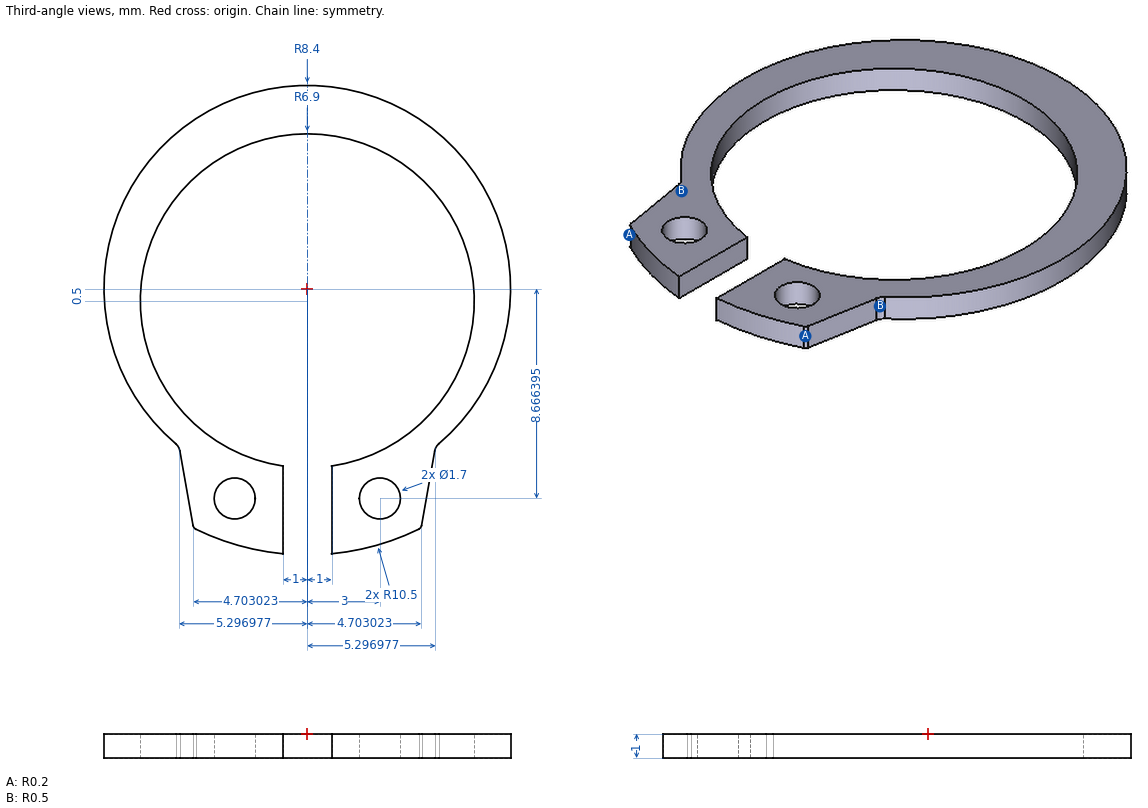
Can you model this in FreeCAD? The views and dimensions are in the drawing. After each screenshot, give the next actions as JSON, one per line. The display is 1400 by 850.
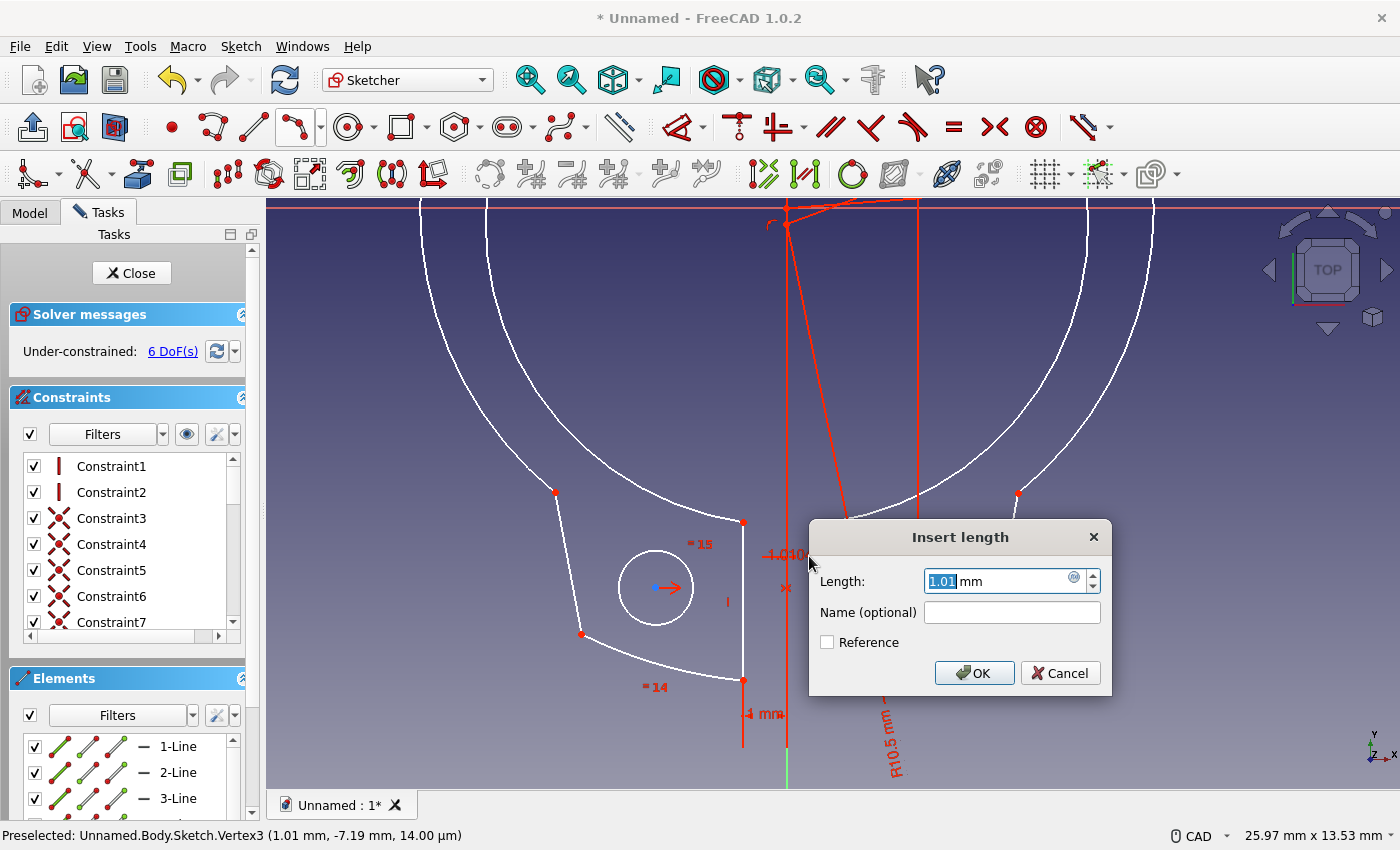
{"action": "type", "text": "1"}
{"action": "key", "text": "Return"}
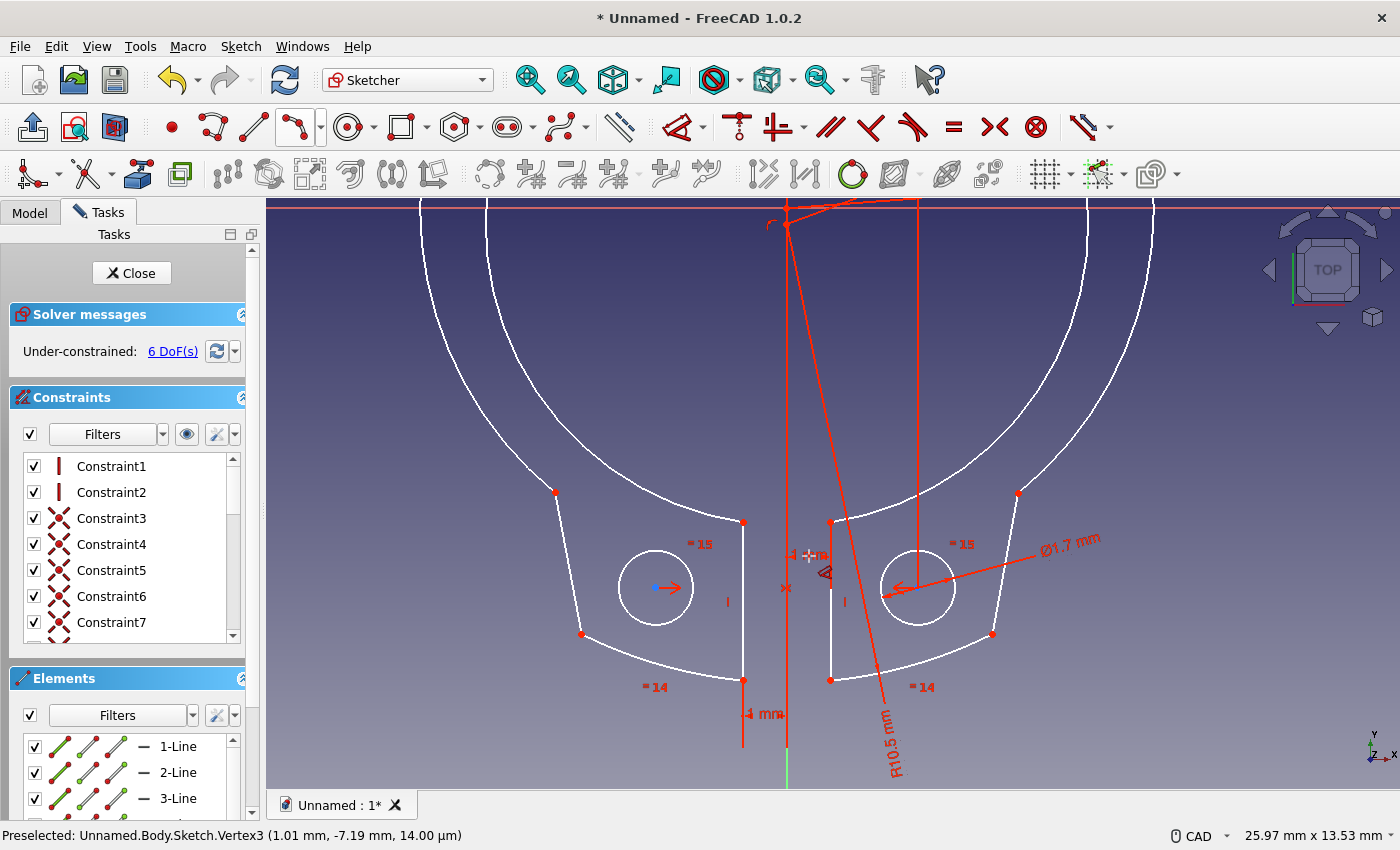
{"action": "scroll", "coordinate": [746, 681], "scroll_direction": "down", "scroll_amount": 4}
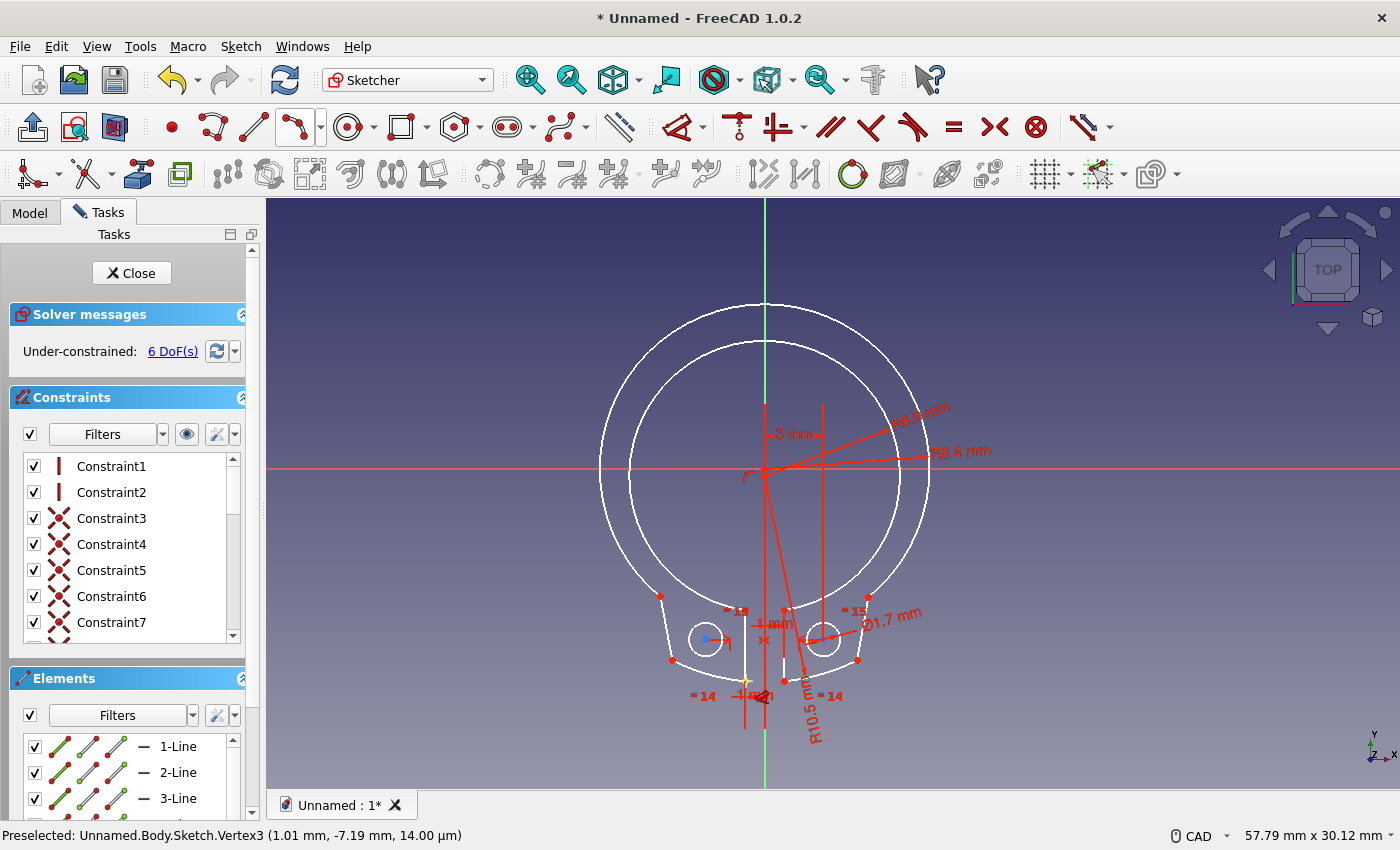
{"action": "scroll", "coordinate": [765, 476], "scroll_direction": "up", "scroll_amount": 7}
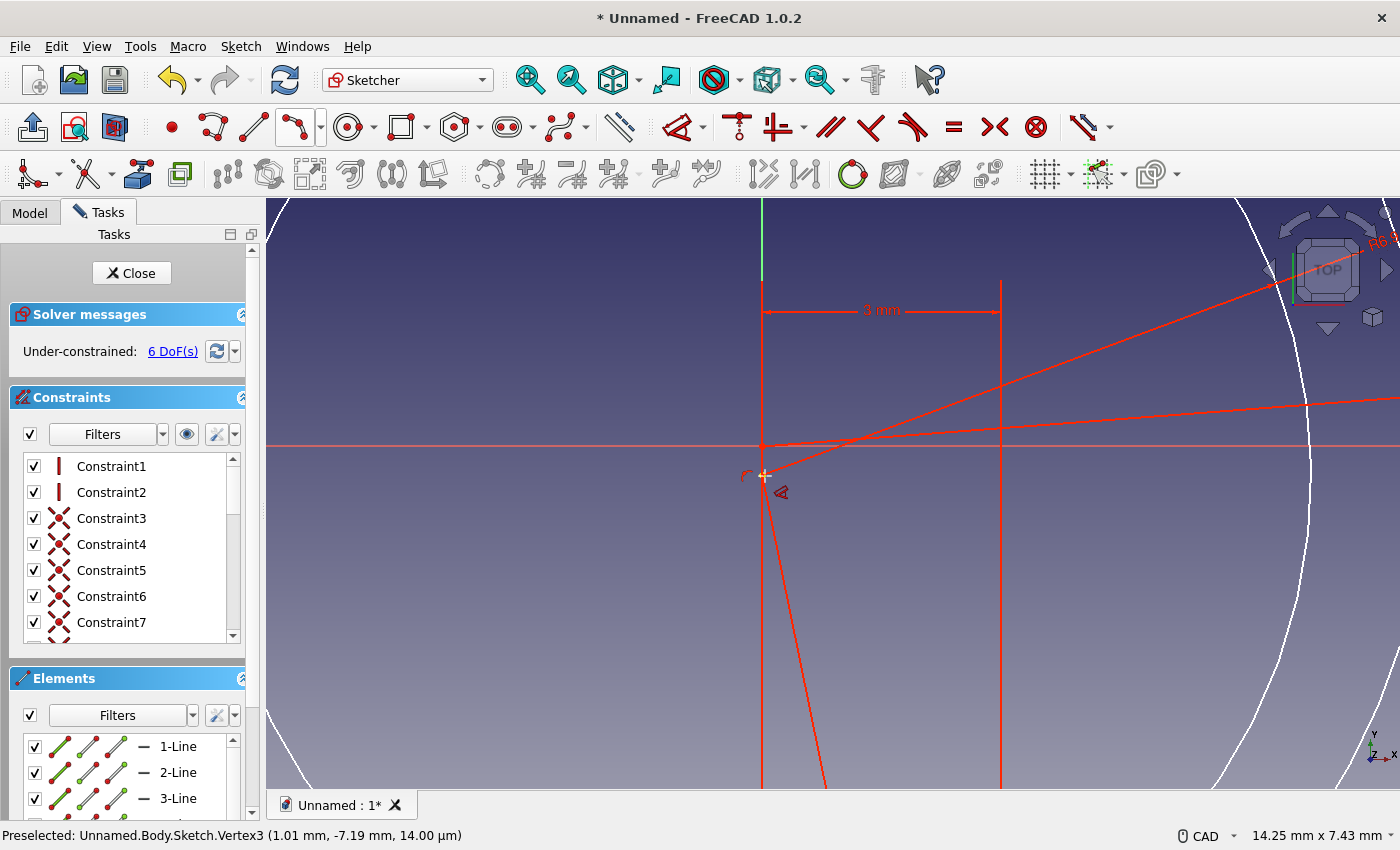
{"action": "left_click", "coordinate": [762, 475]}
{"action": "left_click", "coordinate": [796, 461]}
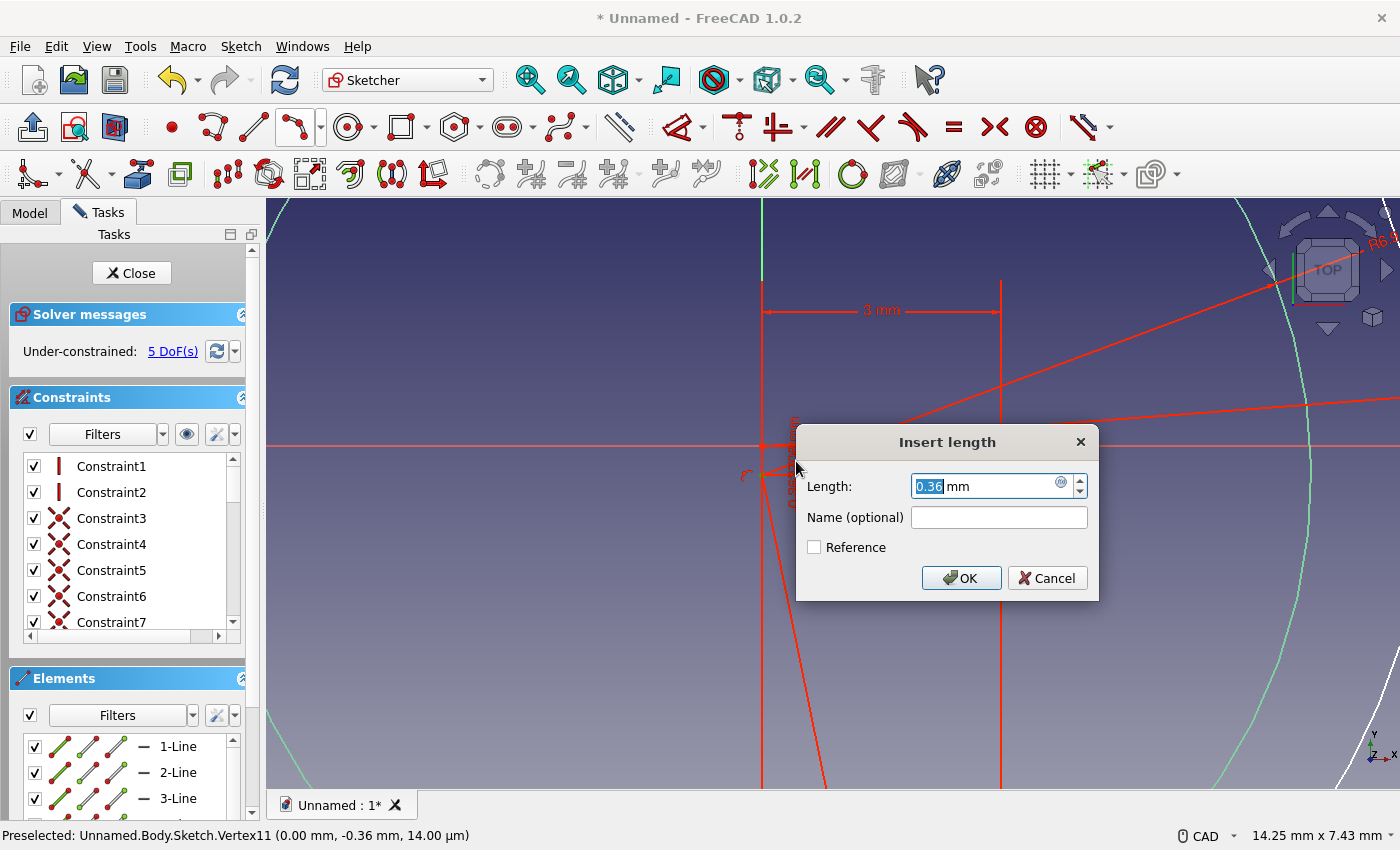
{"action": "type", "text": "0.5"}
{"action": "key", "text": "Return"}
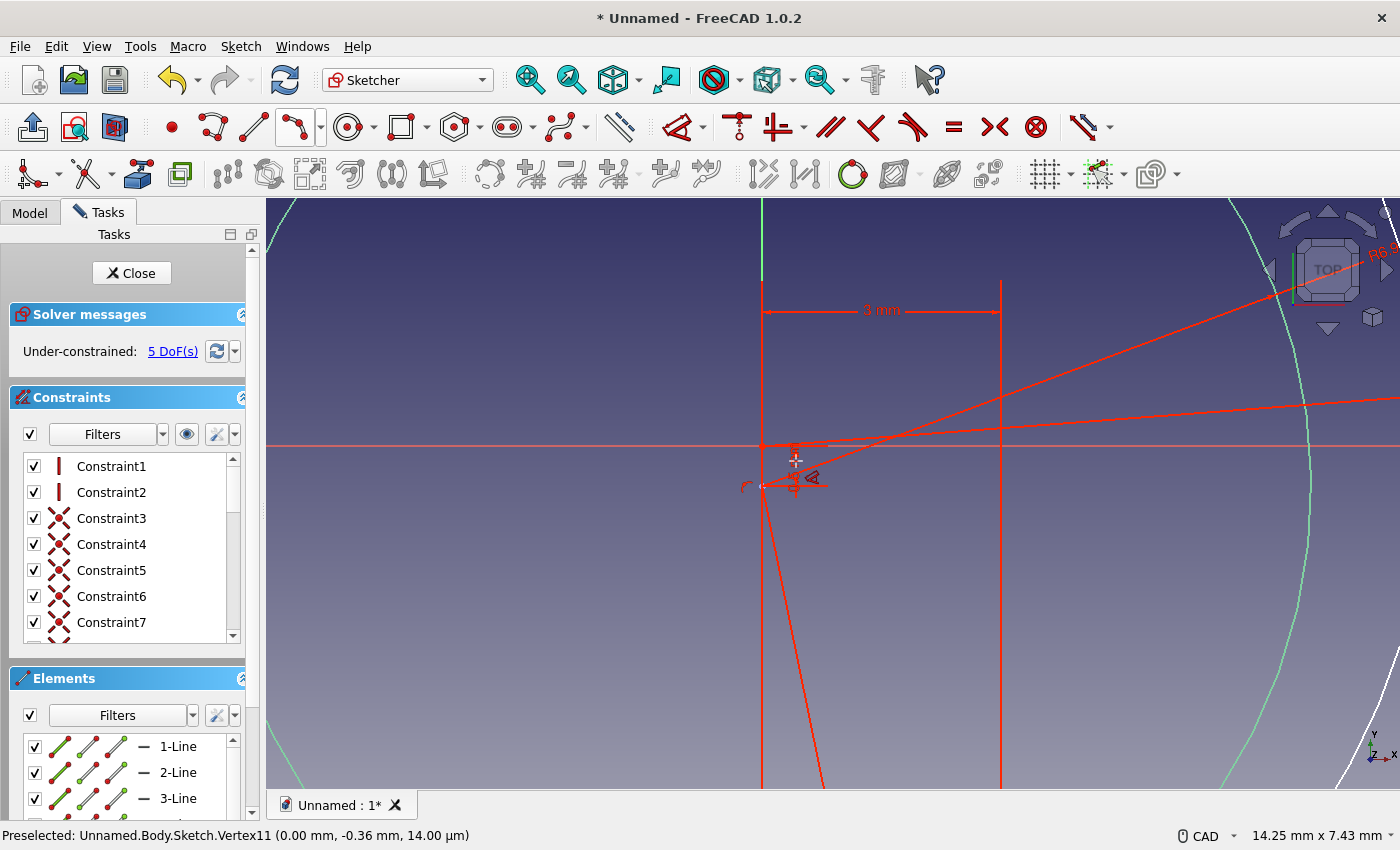
{"action": "scroll", "coordinate": [765, 476], "scroll_direction": "down", "scroll_amount": 7}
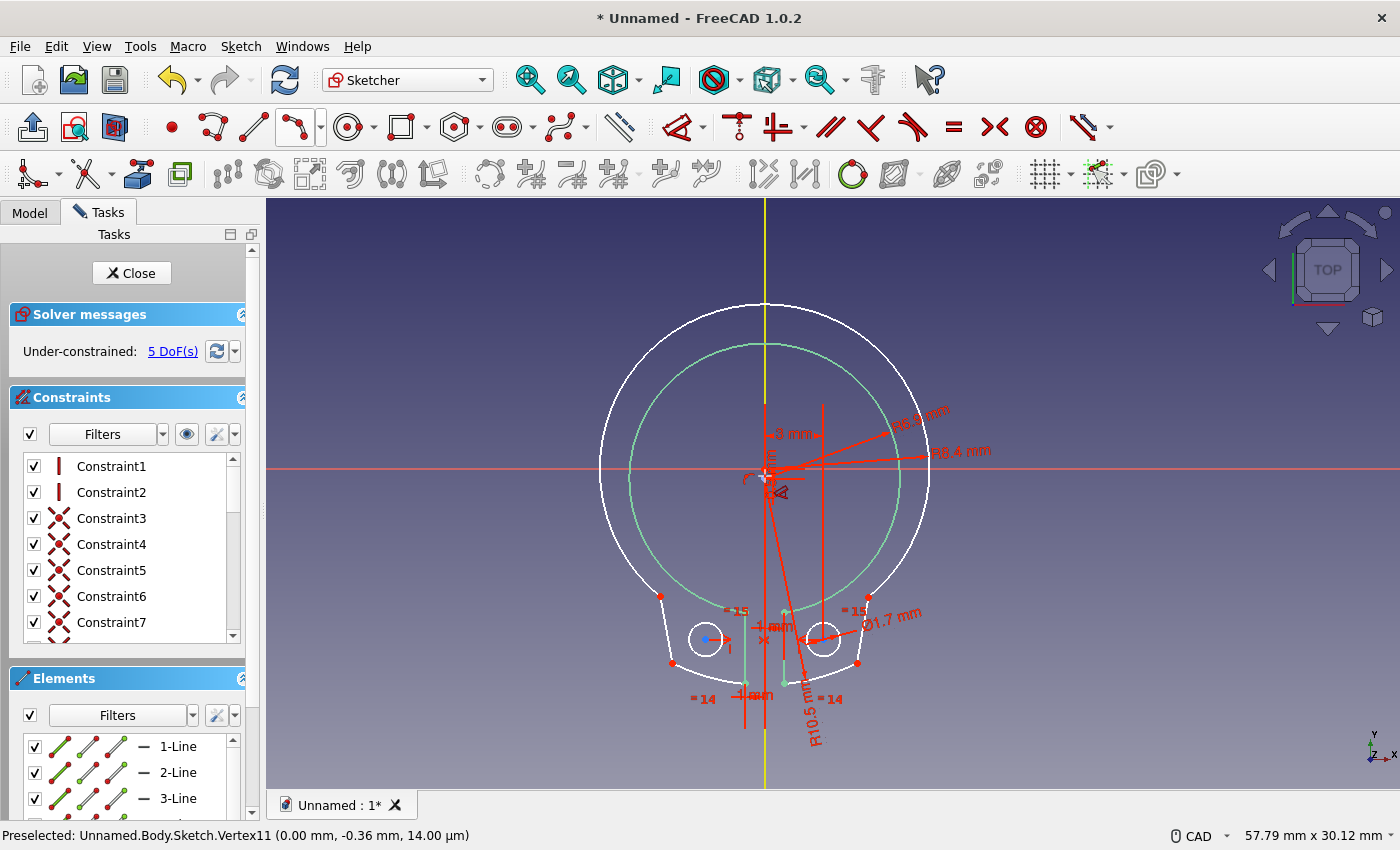
{"action": "left_click", "coordinate": [824, 640]}
{"action": "left_click", "coordinate": [858, 554]}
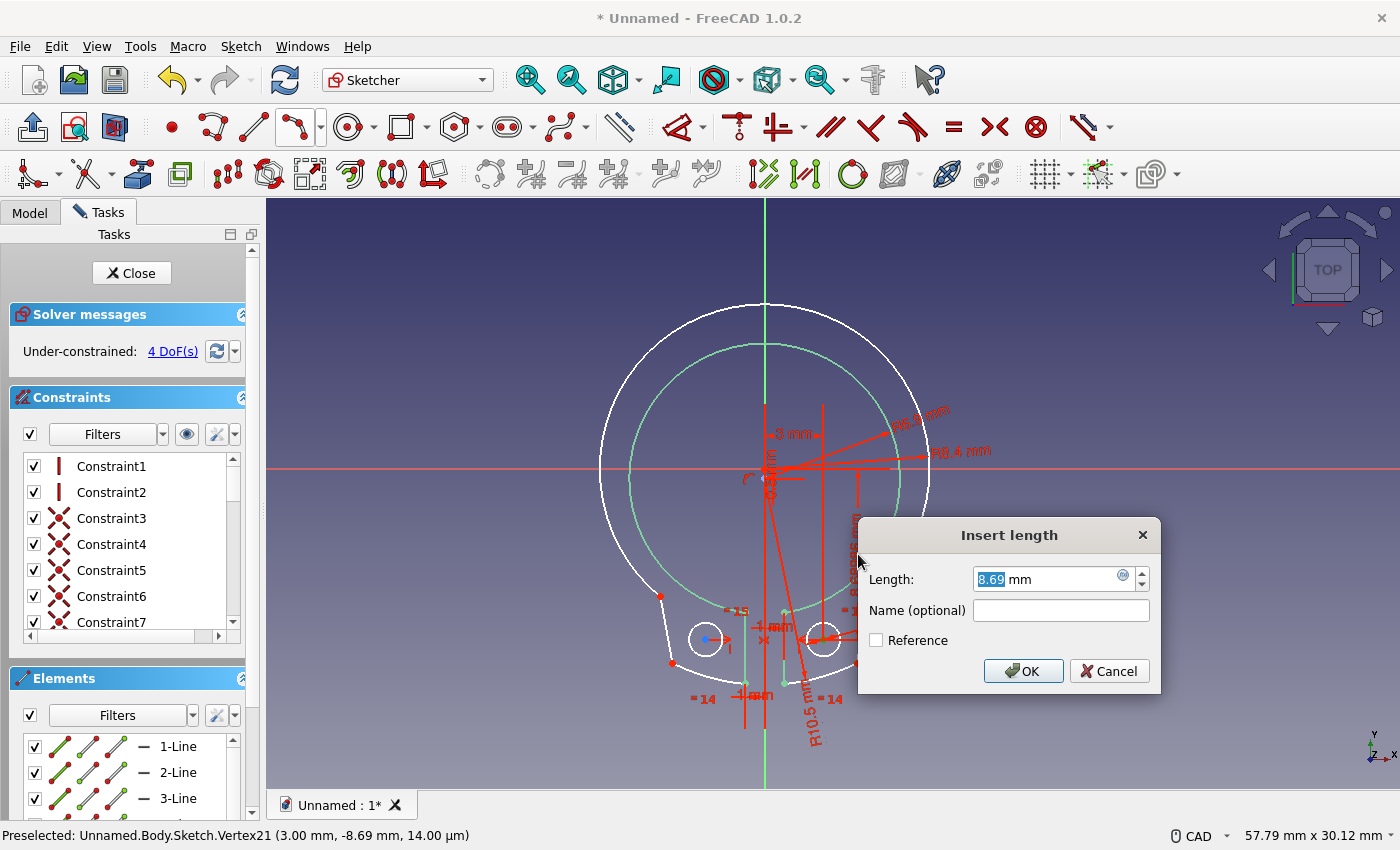
{"action": "type", "text": "8.666395"}
{"action": "key", "text": "Return"}